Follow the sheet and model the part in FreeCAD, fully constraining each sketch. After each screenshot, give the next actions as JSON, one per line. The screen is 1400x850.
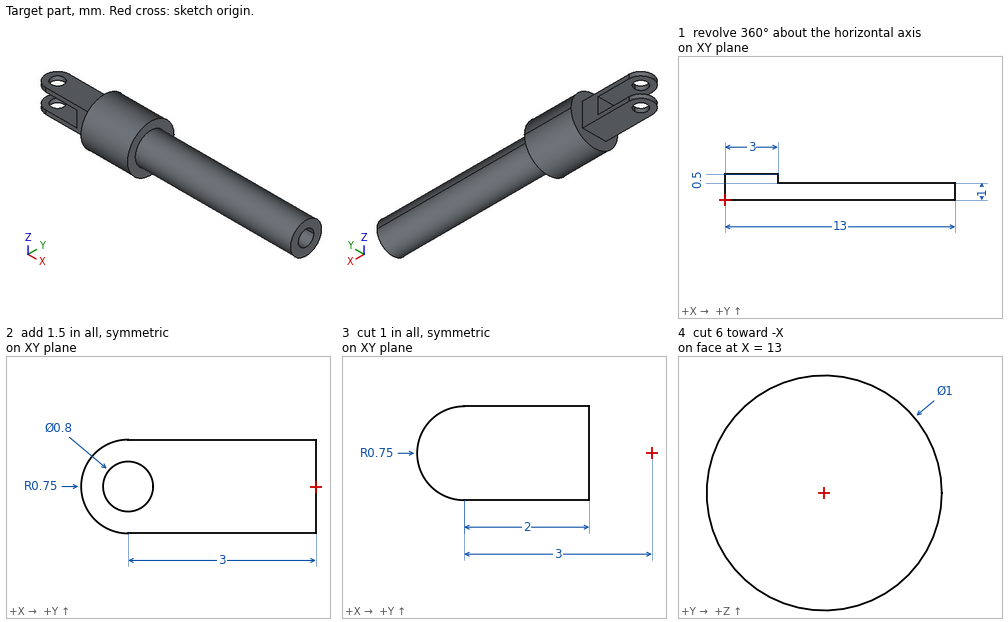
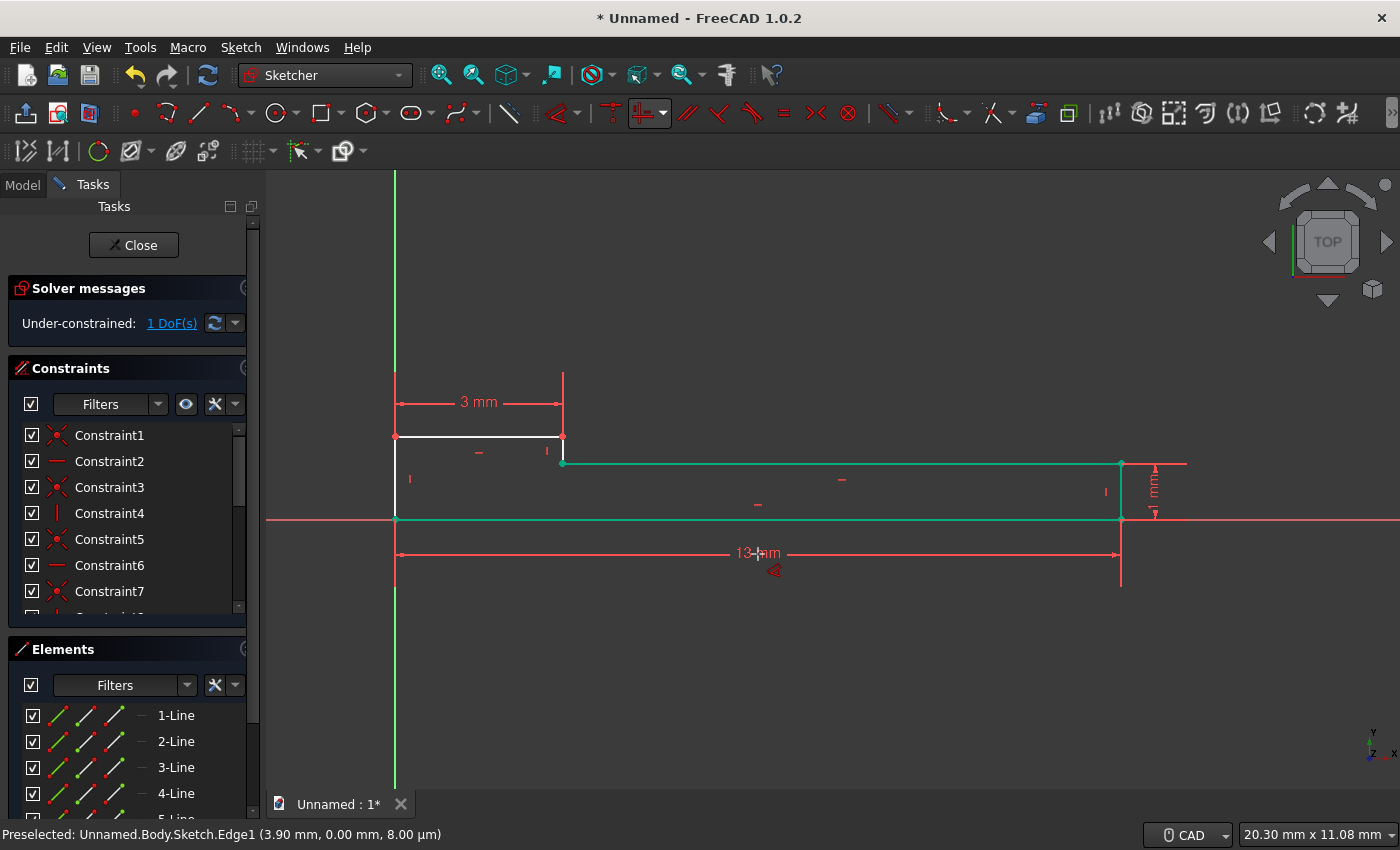
{"action": "scroll", "coordinate": [563, 453], "scroll_direction": "up", "scroll_amount": 2}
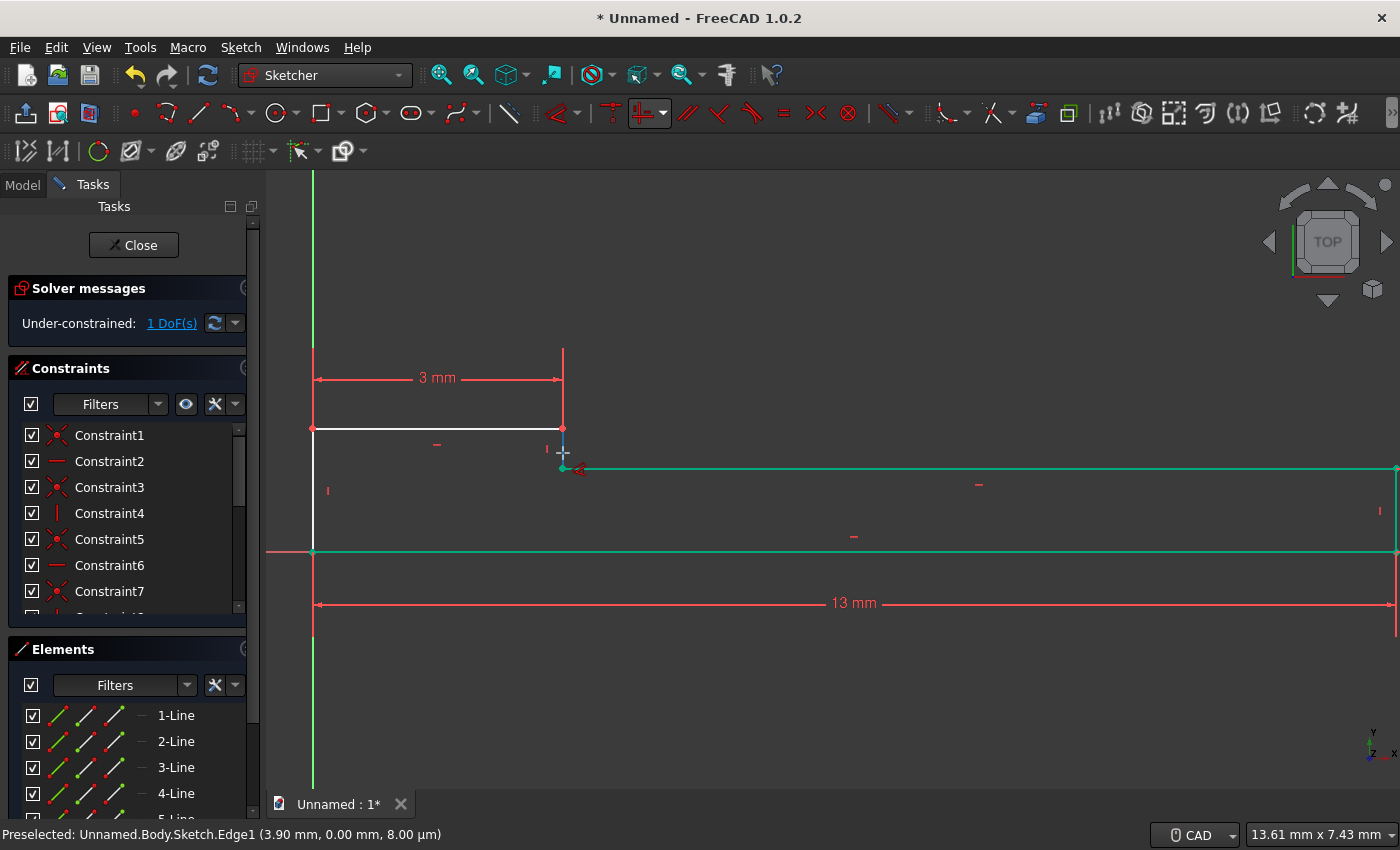
{"action": "left_click", "coordinate": [563, 453]}
{"action": "left_click", "coordinate": [529, 449]}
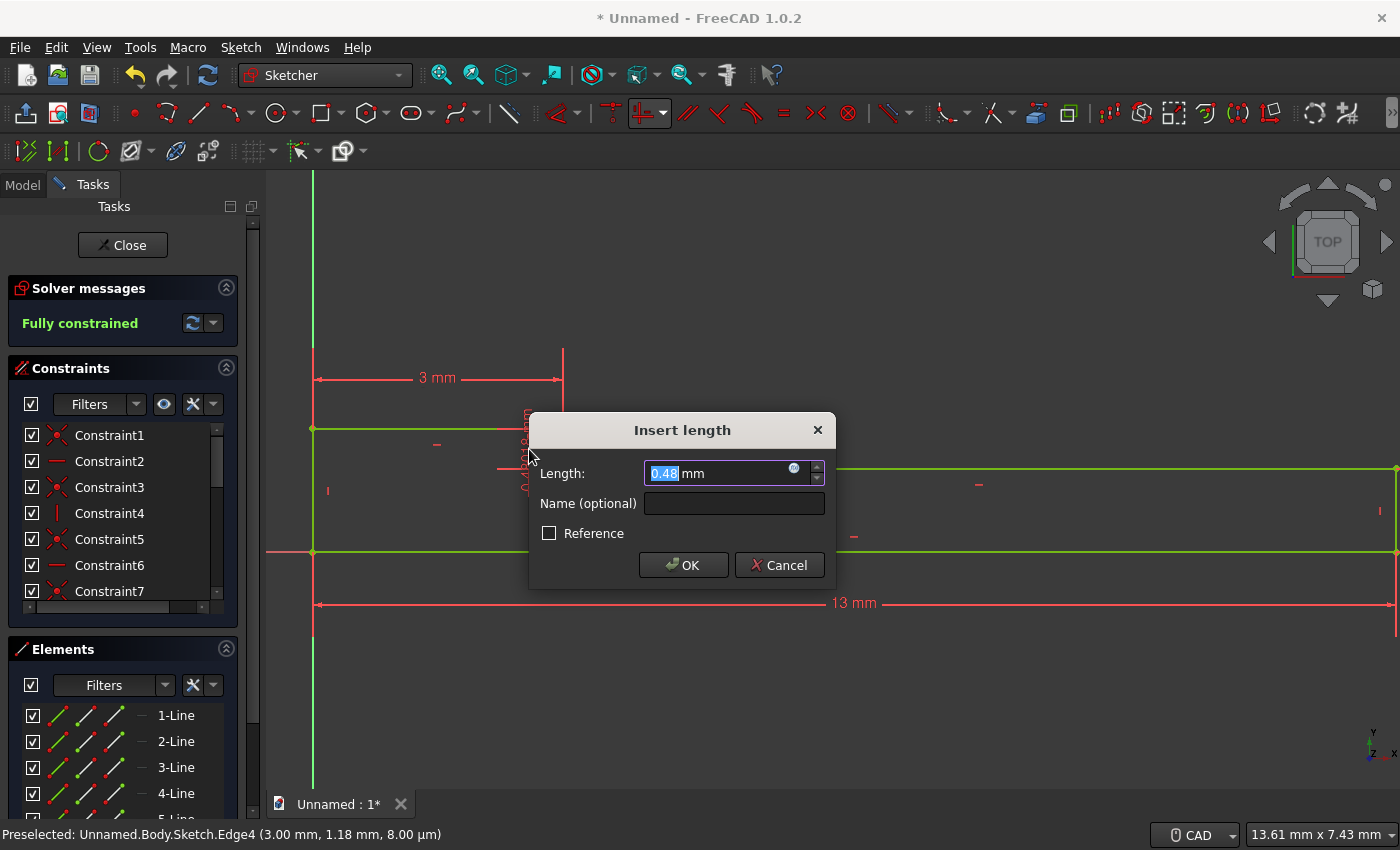
{"action": "type", "text": "0.5"}
{"action": "key", "text": "Return"}
{"action": "key", "text": "Escape"}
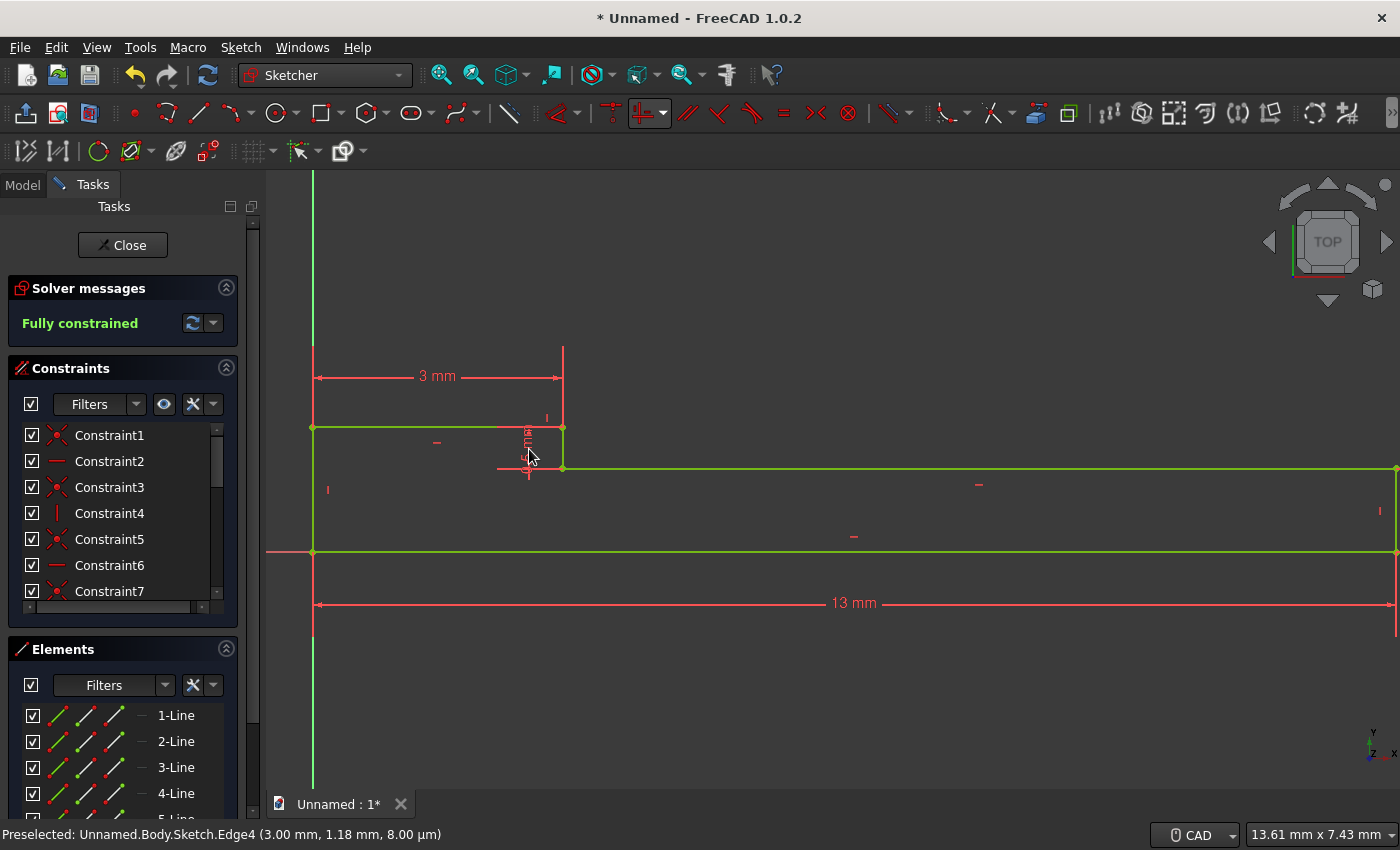
{"action": "left_click", "coordinate": [123, 245]}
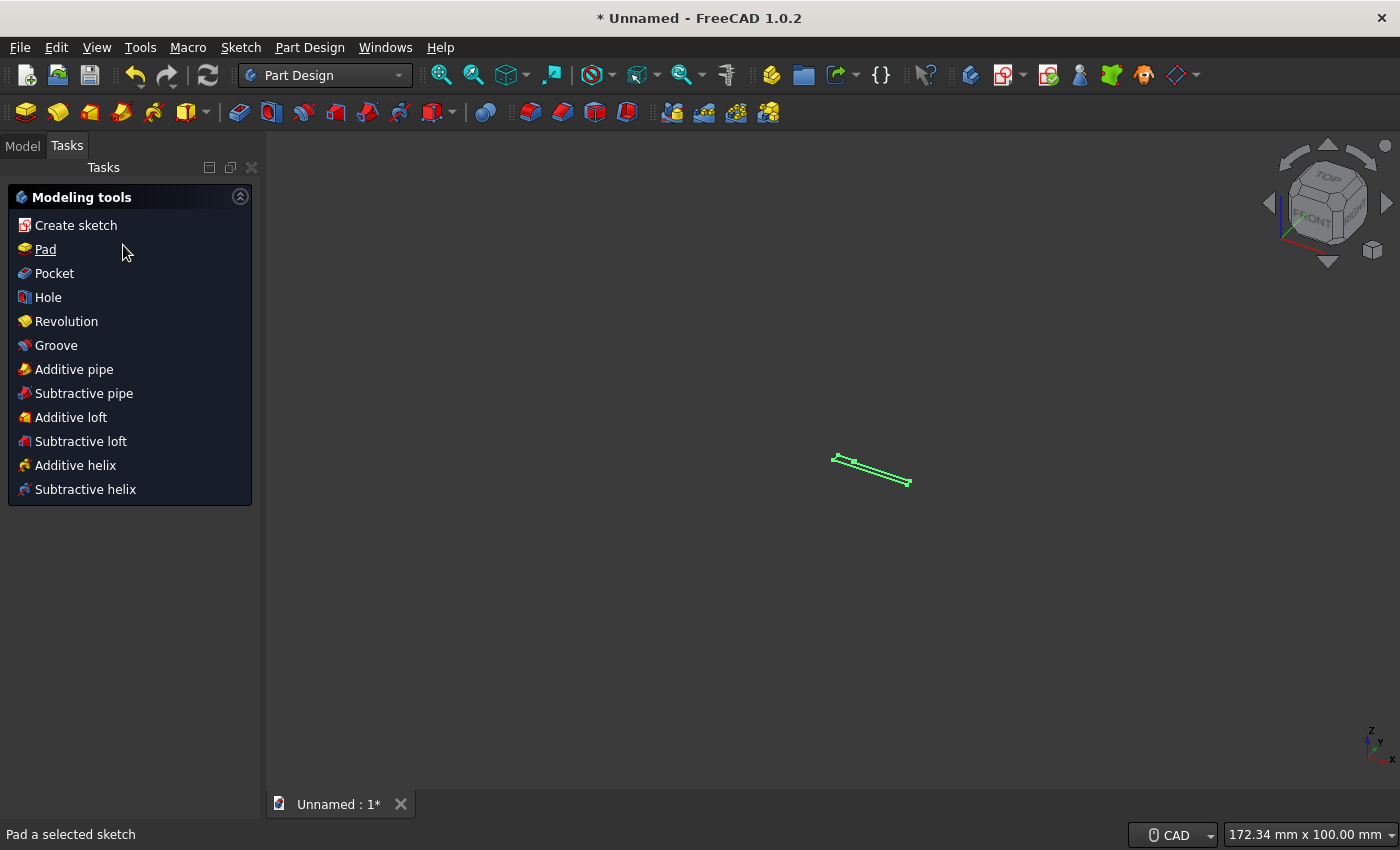
{"action": "left_click", "coordinate": [58, 112]}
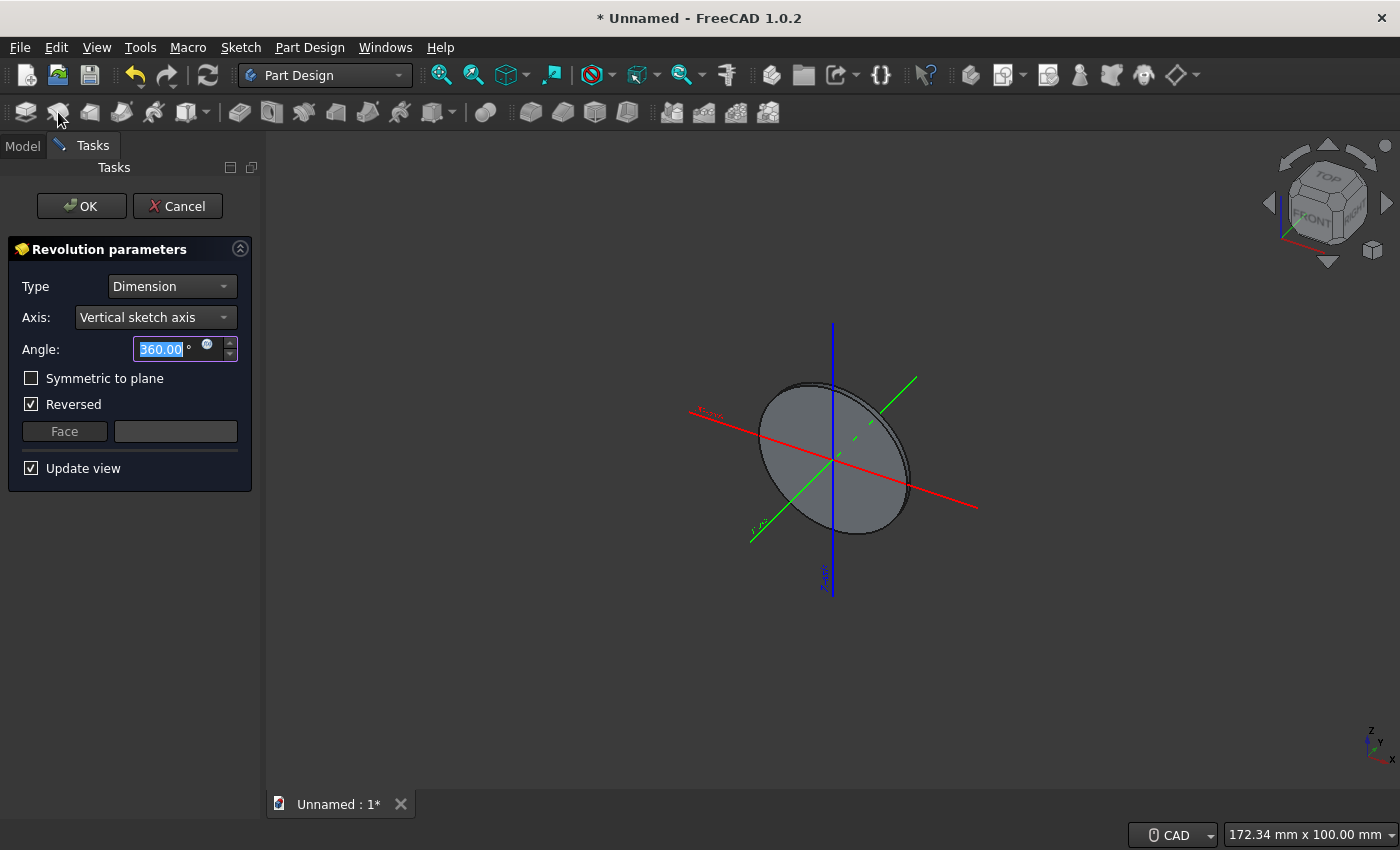
{"action": "left_click", "coordinate": [156, 318]}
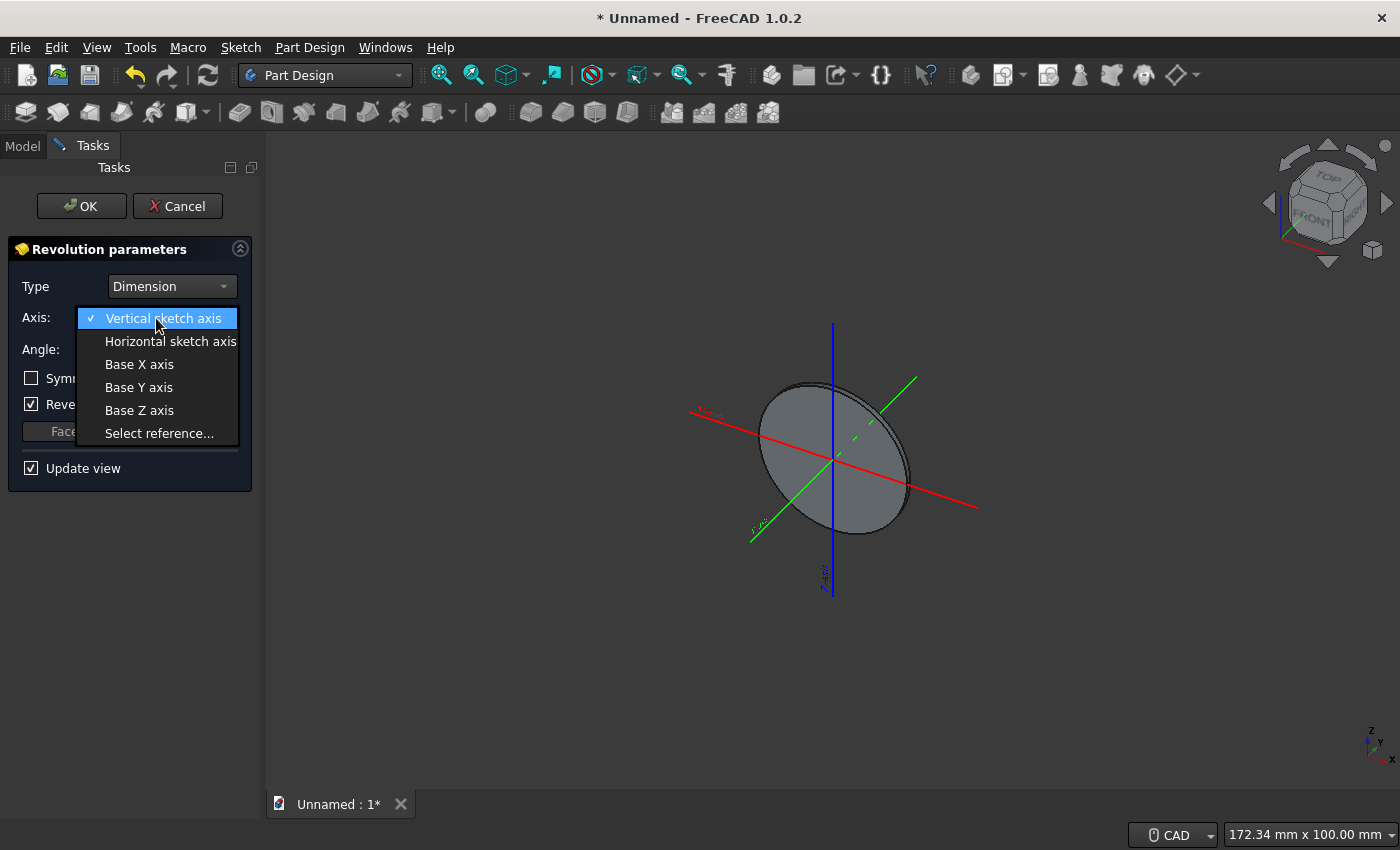
{"action": "left_click", "coordinate": [156, 342]}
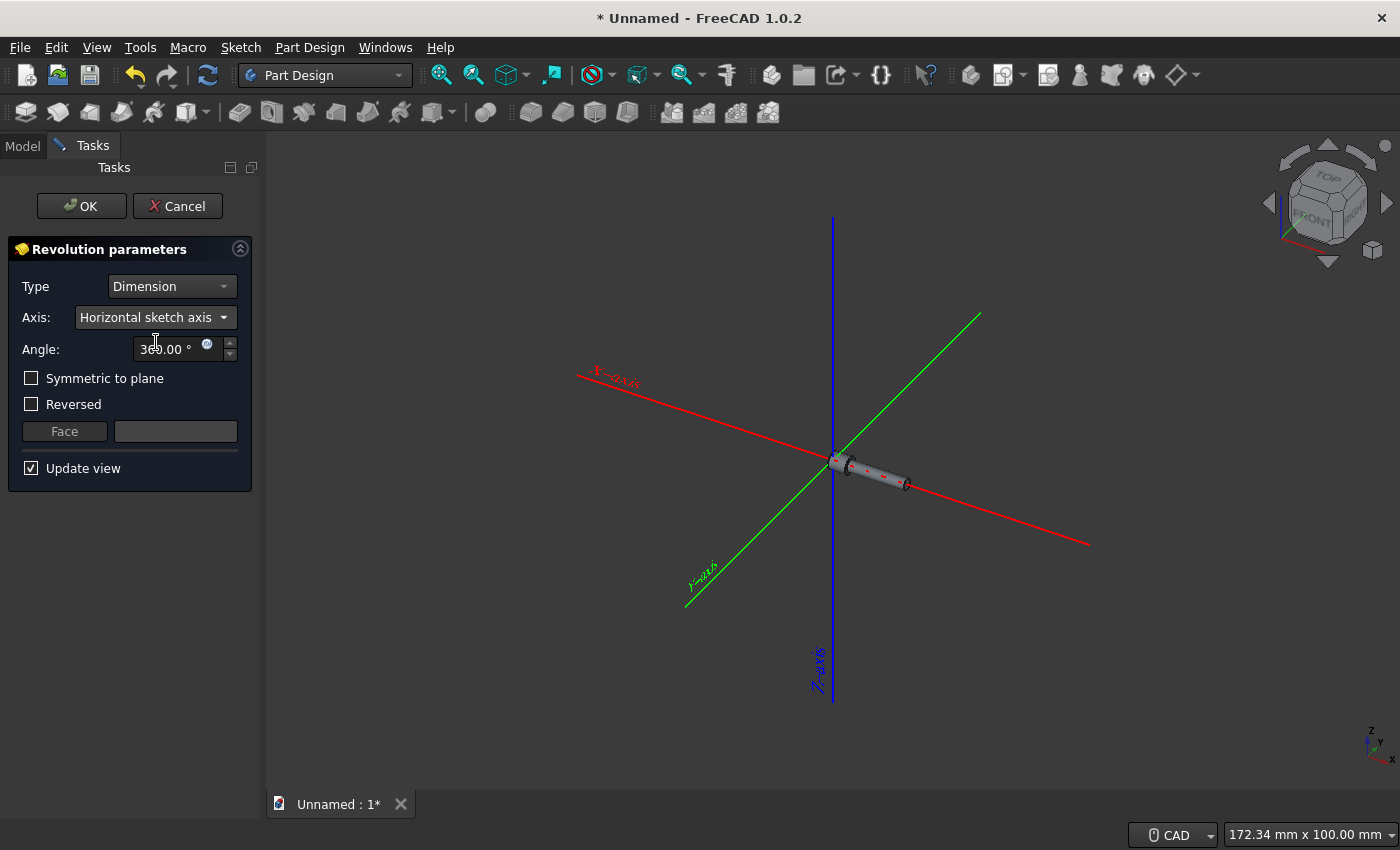
{"action": "left_click", "coordinate": [82, 206]}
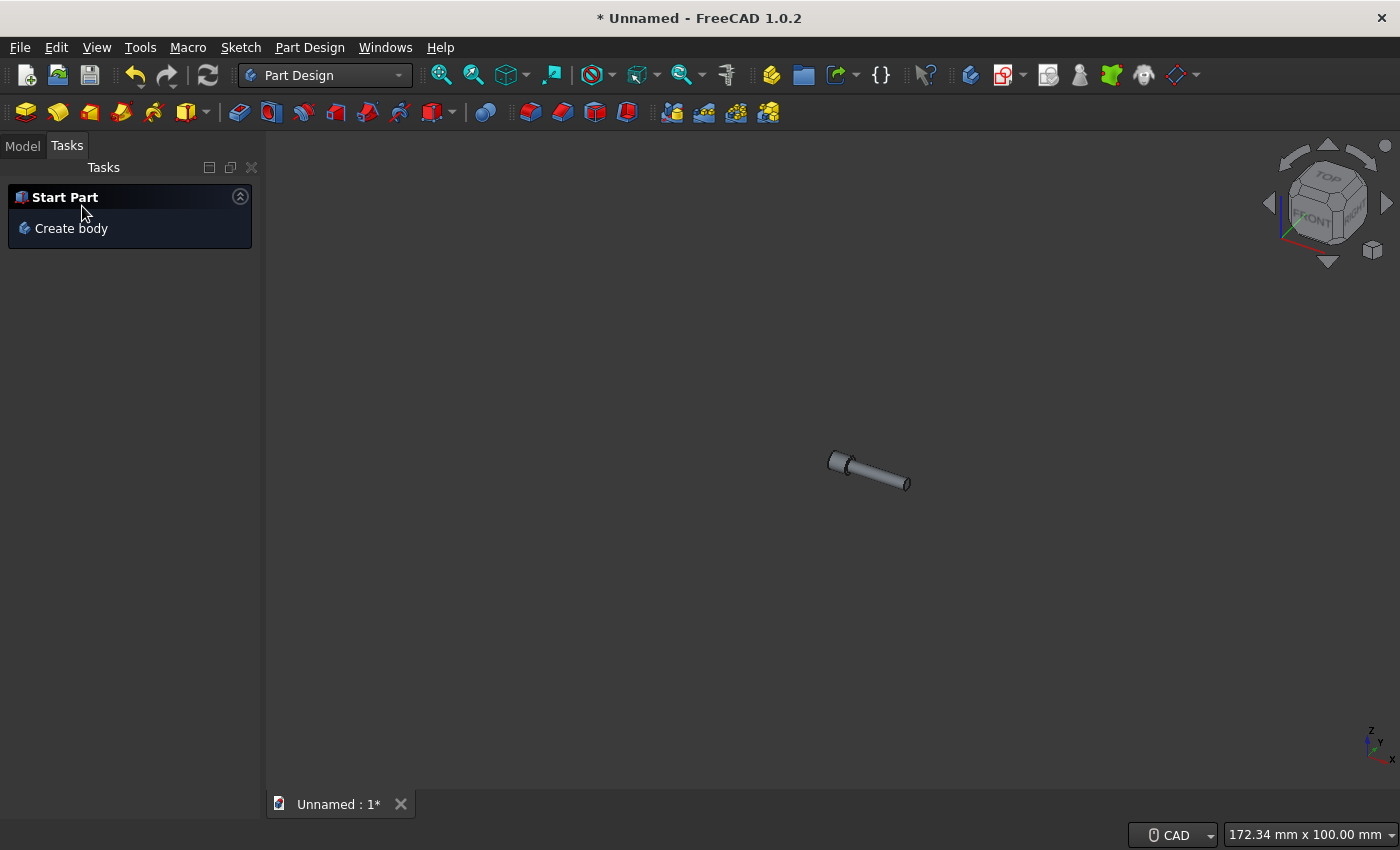
{"action": "left_click", "coordinate": [442, 76]}